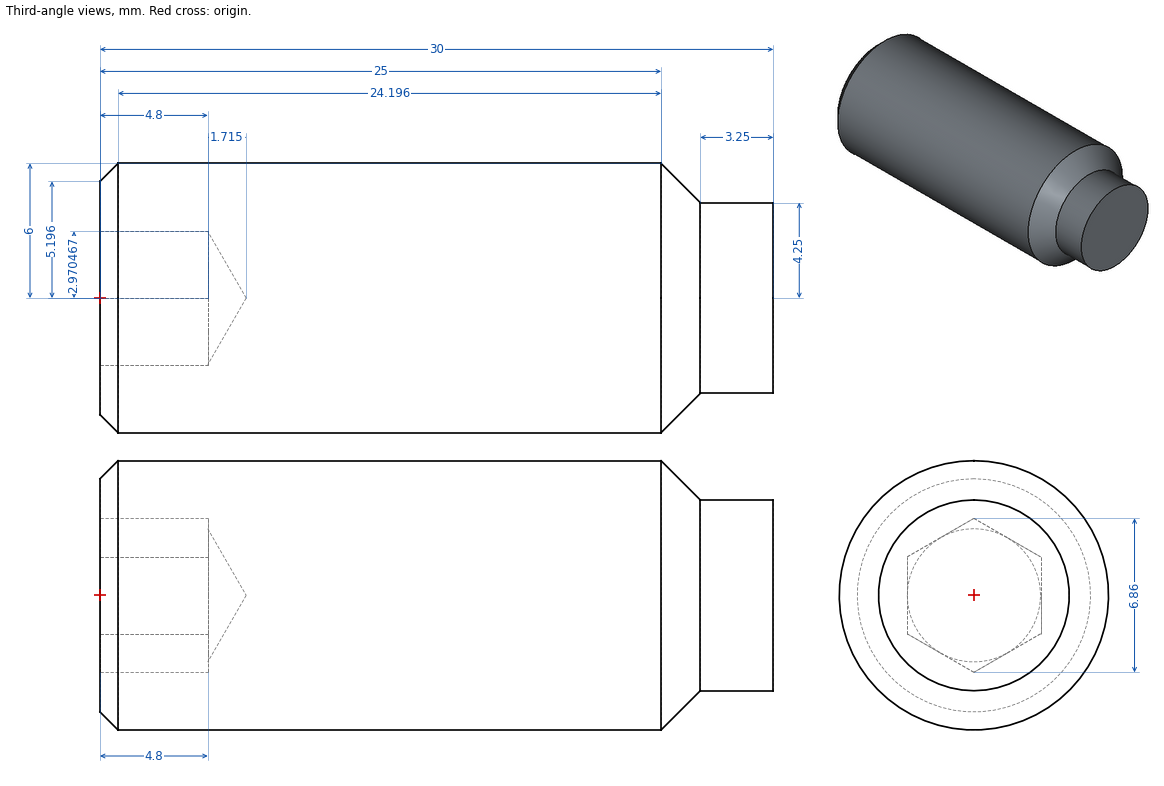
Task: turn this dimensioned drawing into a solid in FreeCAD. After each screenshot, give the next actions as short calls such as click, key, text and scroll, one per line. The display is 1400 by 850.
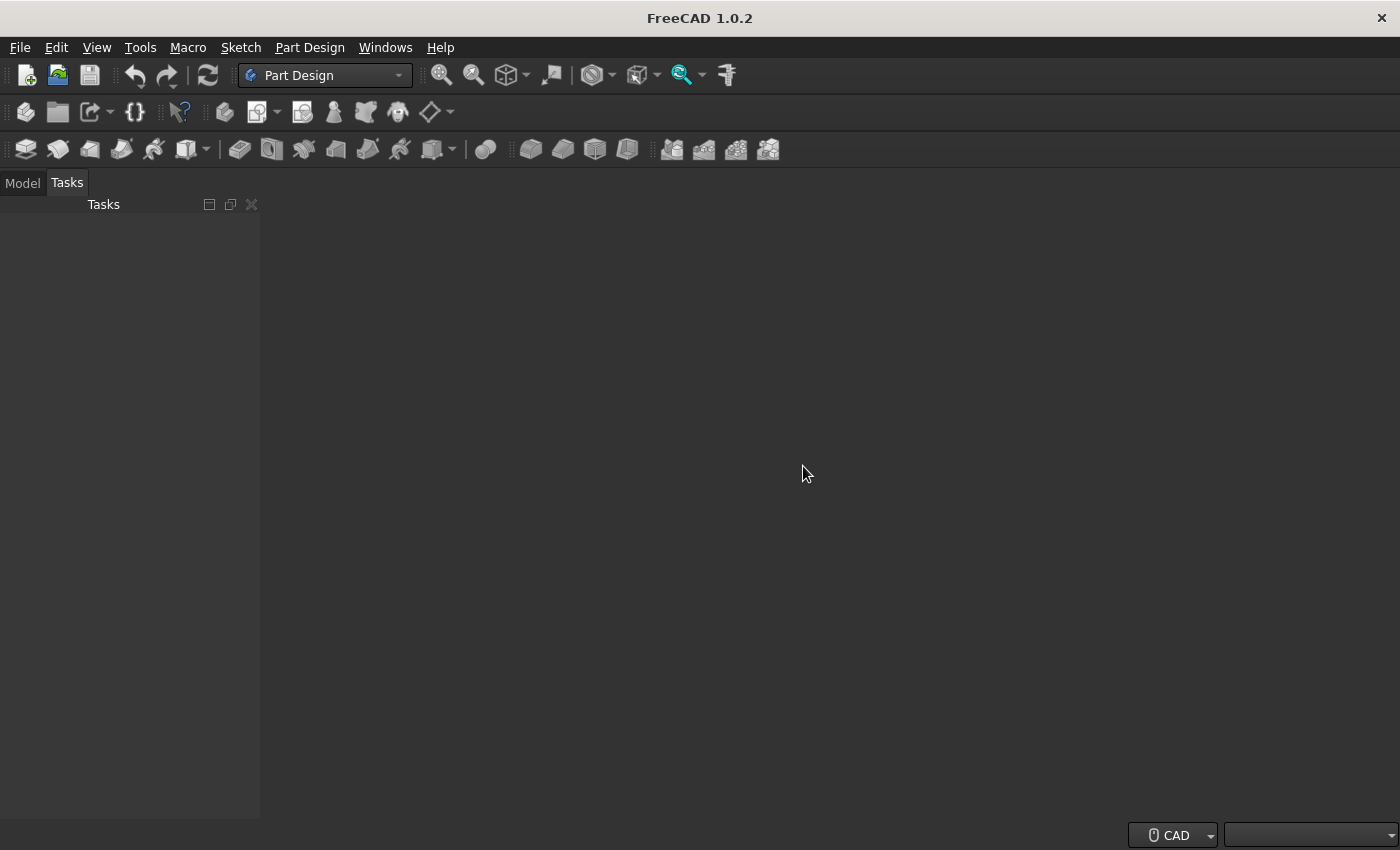
click(26, 76)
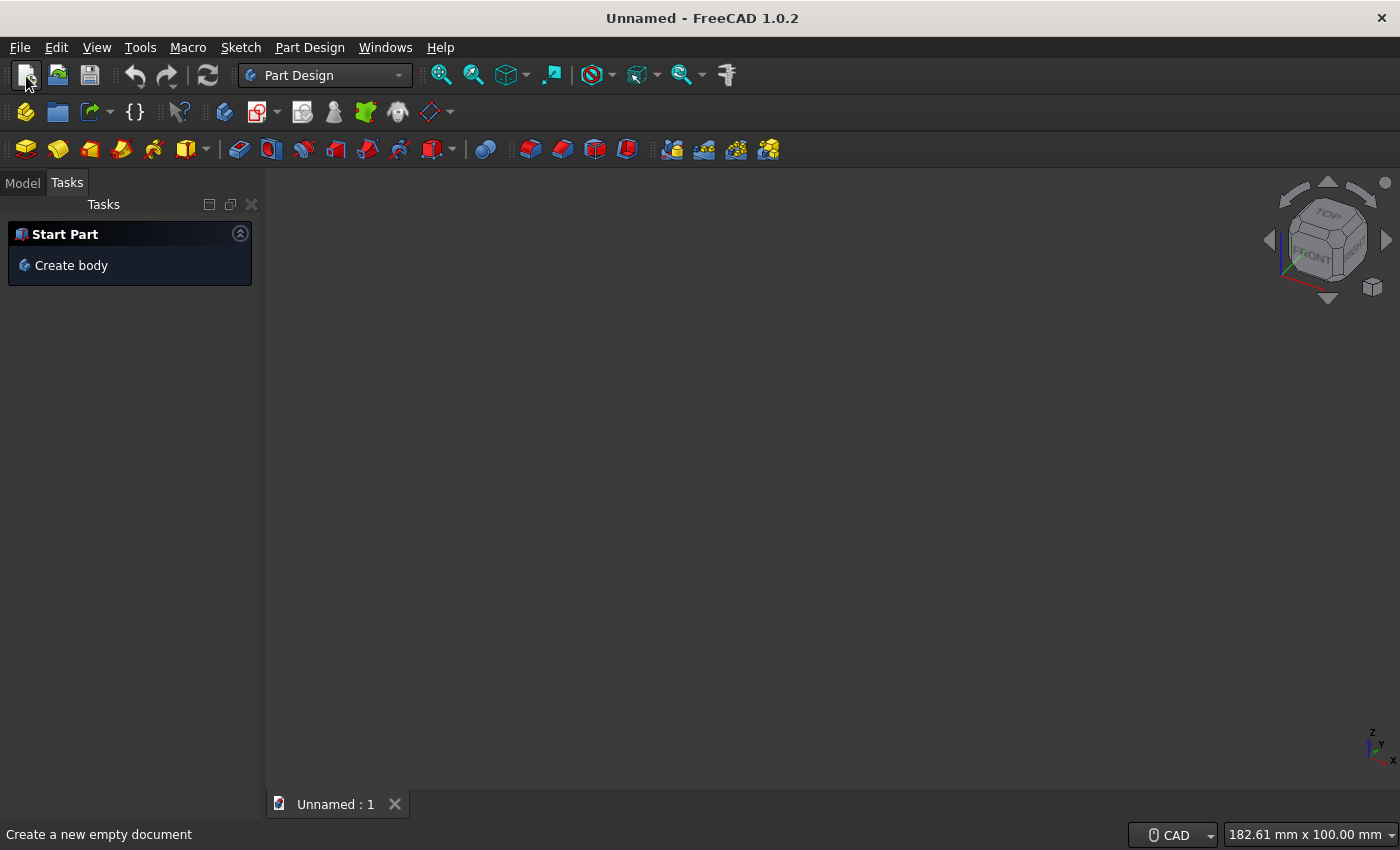
click(258, 112)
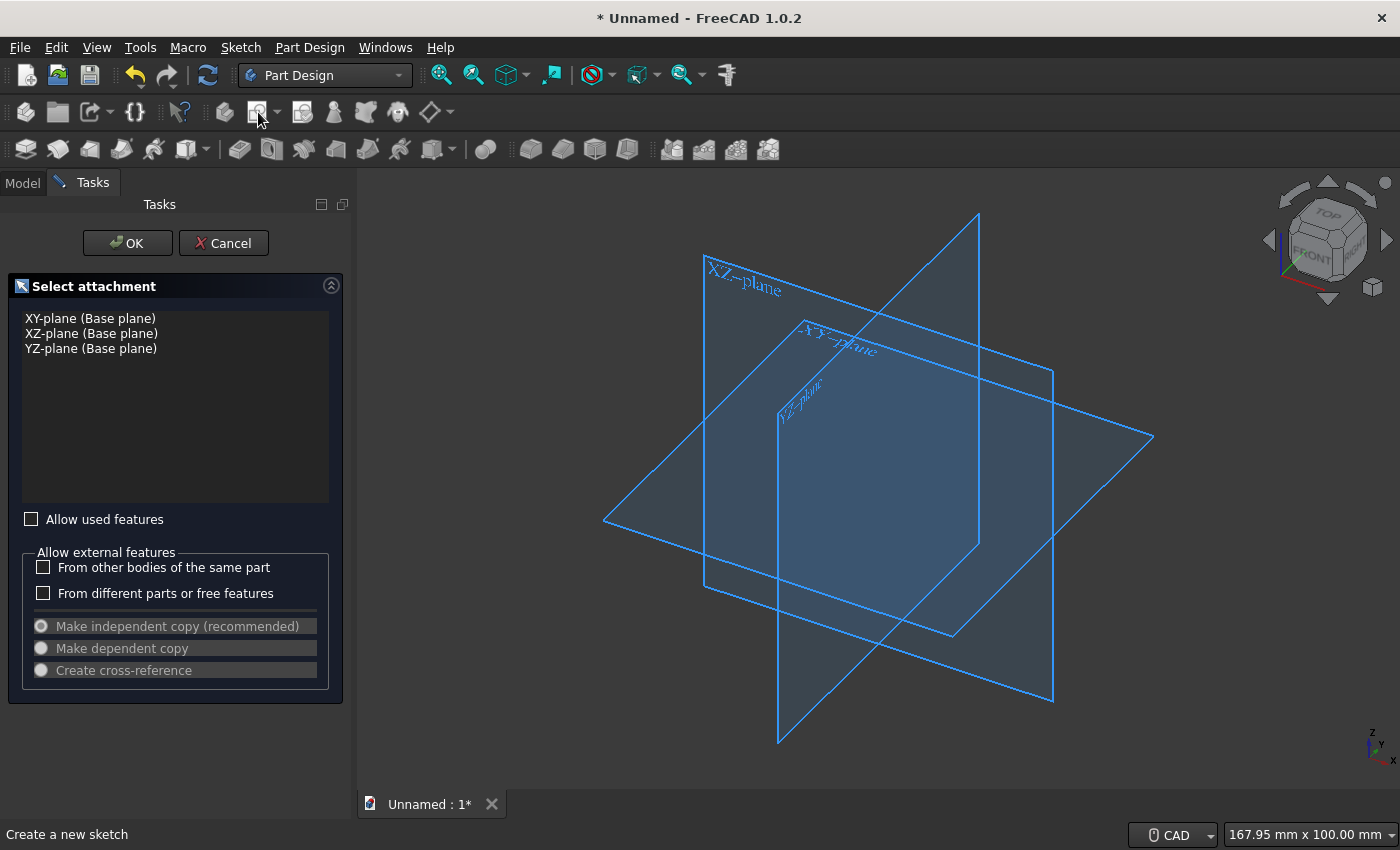
click(82, 318)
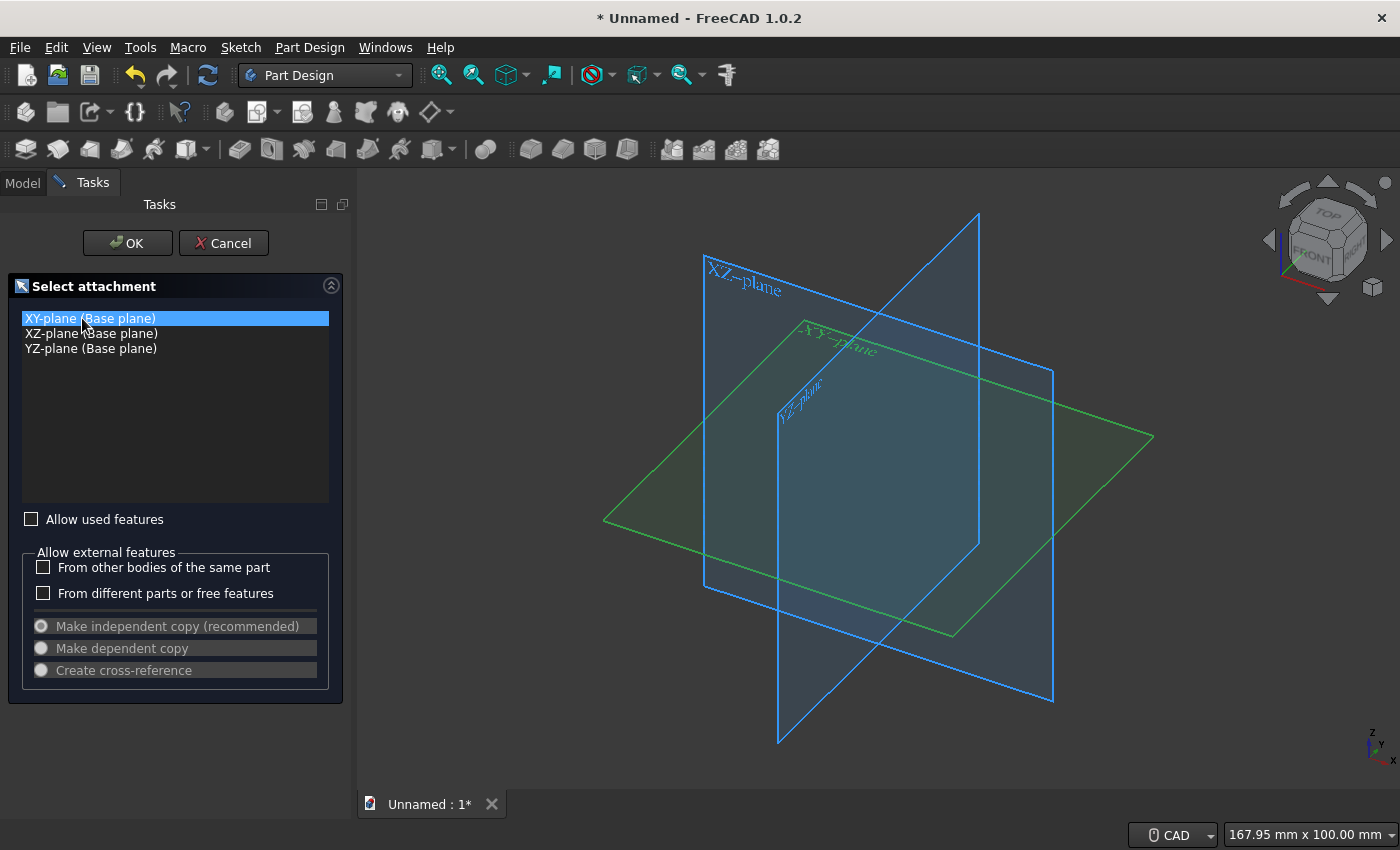
click(128, 243)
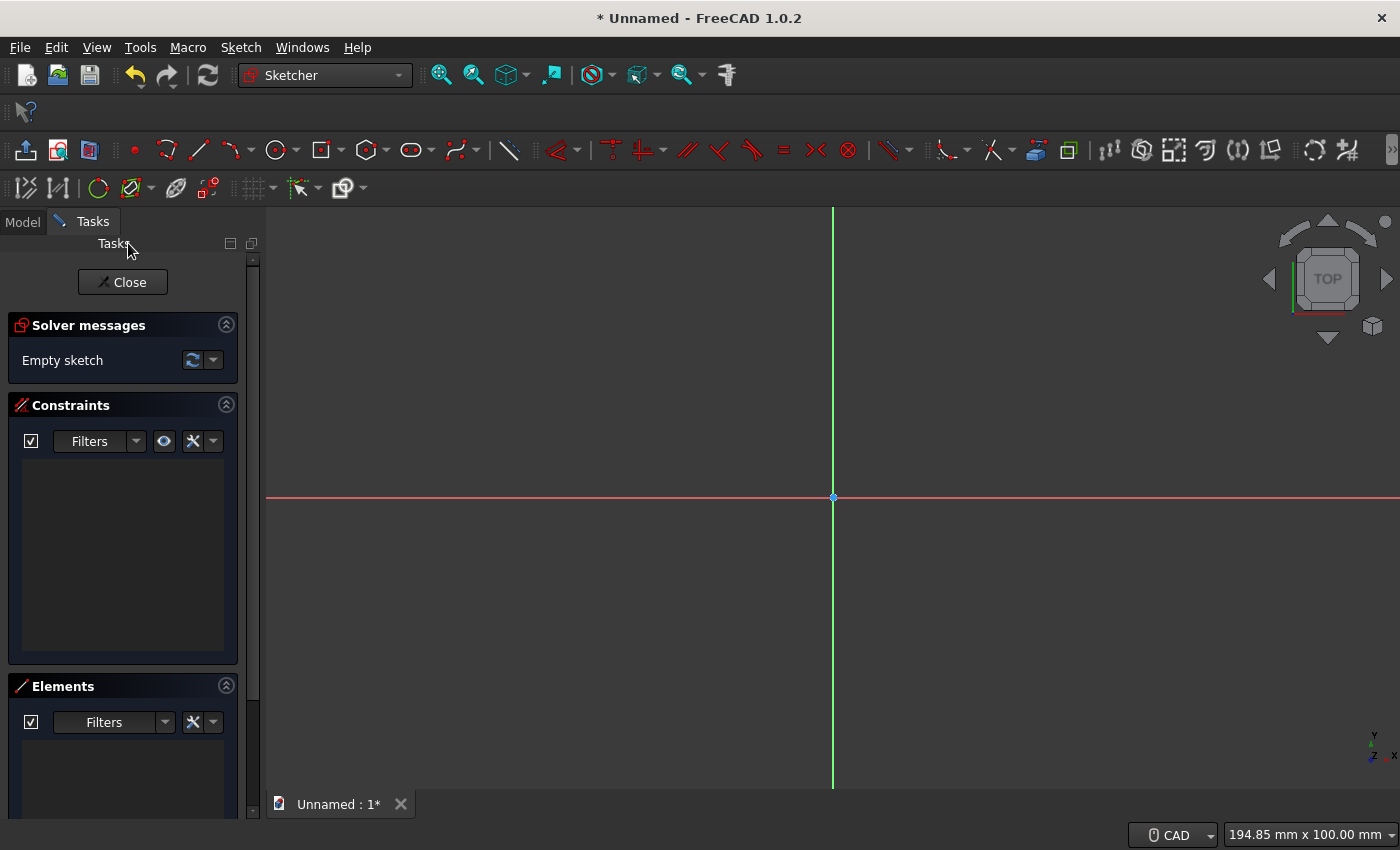
scroll(971, 475, up, 7)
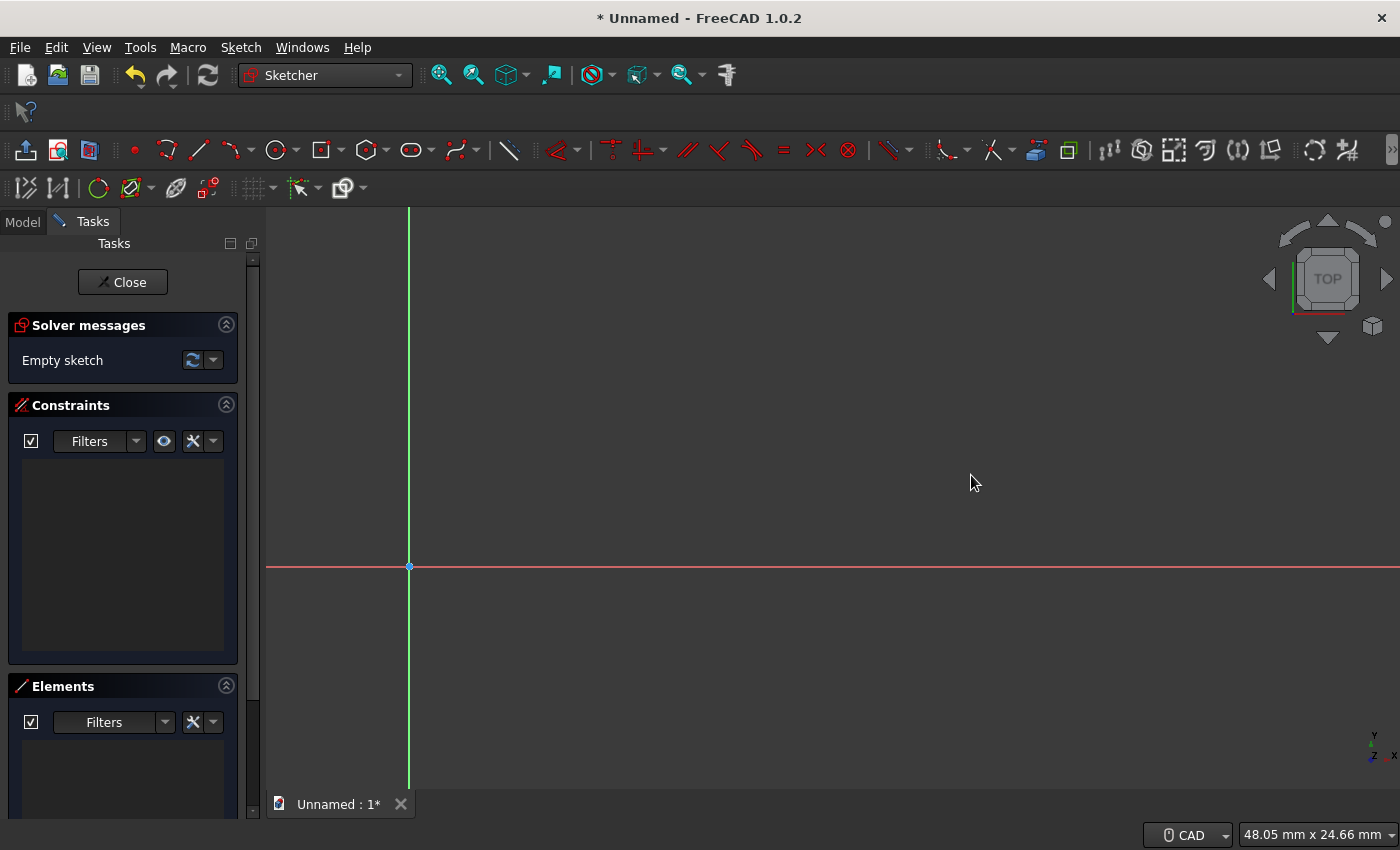
click(168, 150)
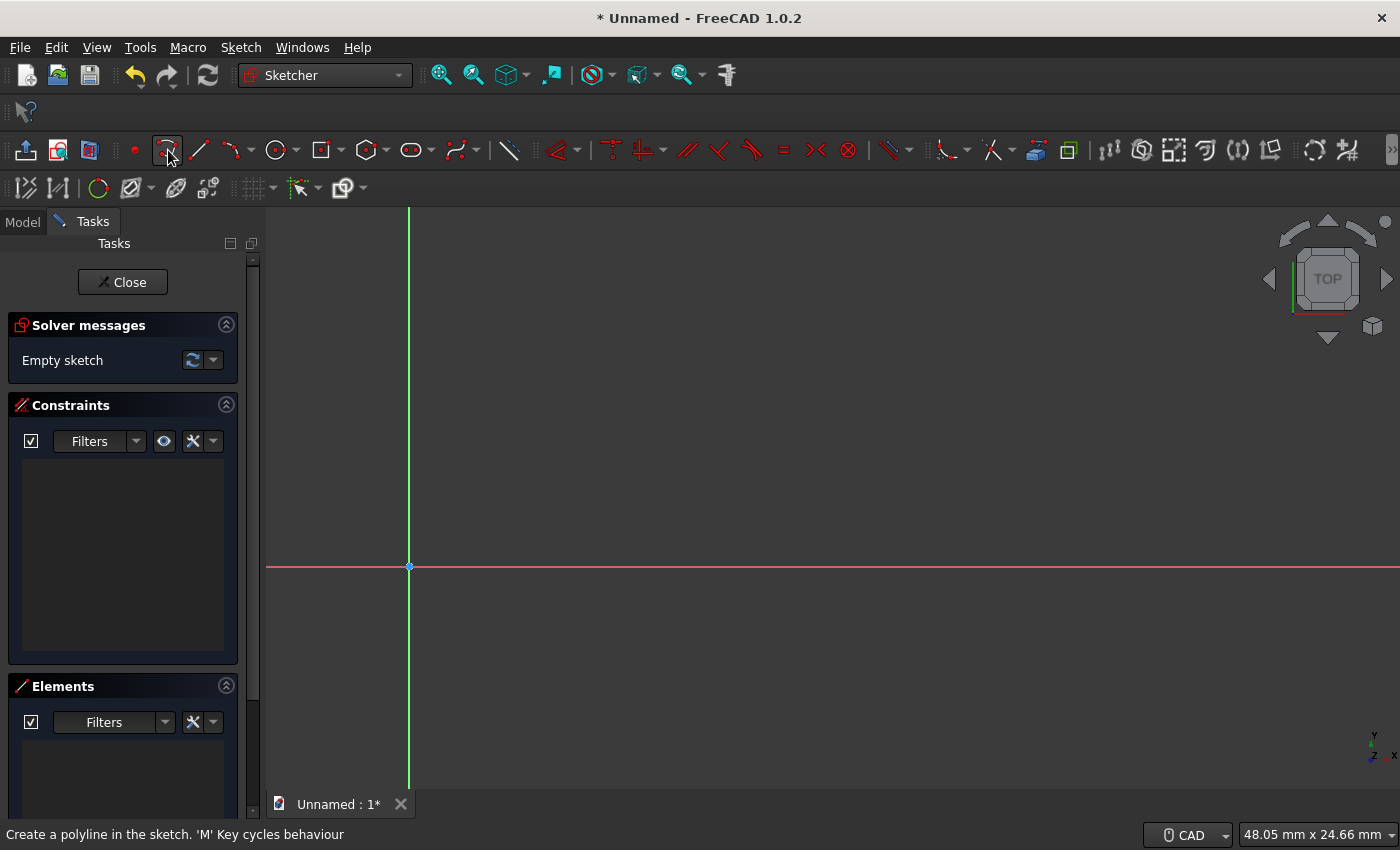
click(409, 567)
click(1118, 558)
click(1118, 467)
click(1041, 467)
click(1000, 425)
click(428, 425)
click(418, 444)
click(409, 567)
key(Escape)
key(Escape)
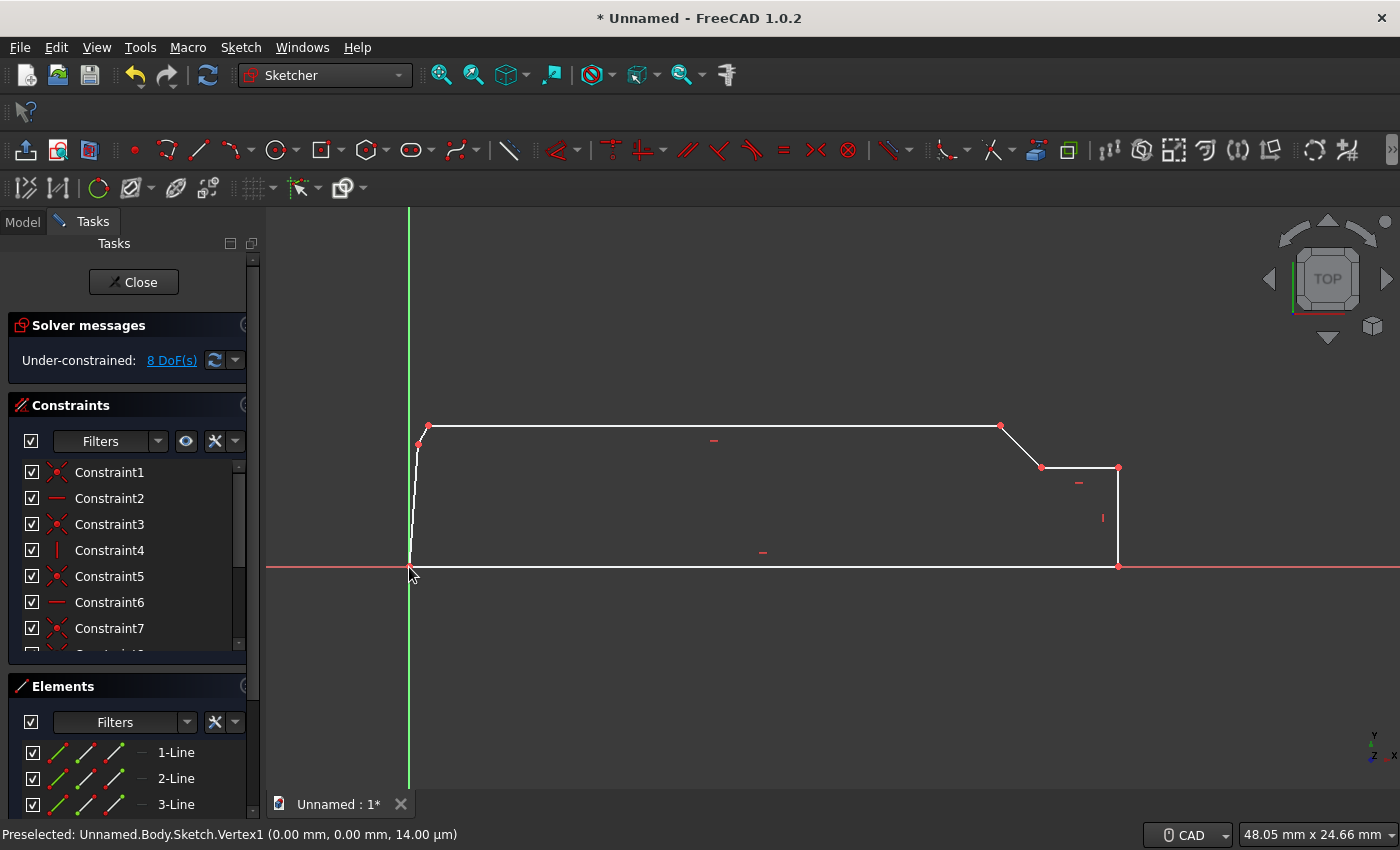
click(412, 530)